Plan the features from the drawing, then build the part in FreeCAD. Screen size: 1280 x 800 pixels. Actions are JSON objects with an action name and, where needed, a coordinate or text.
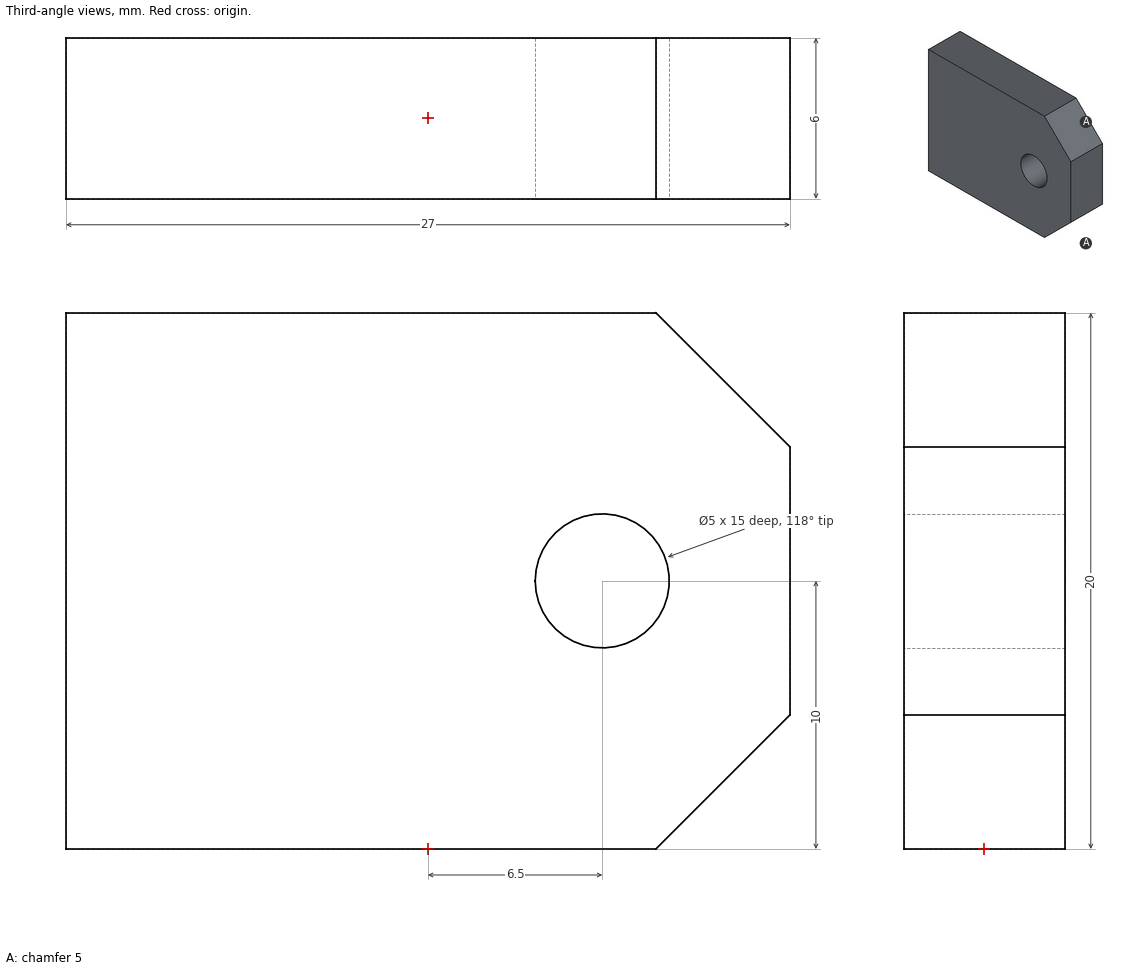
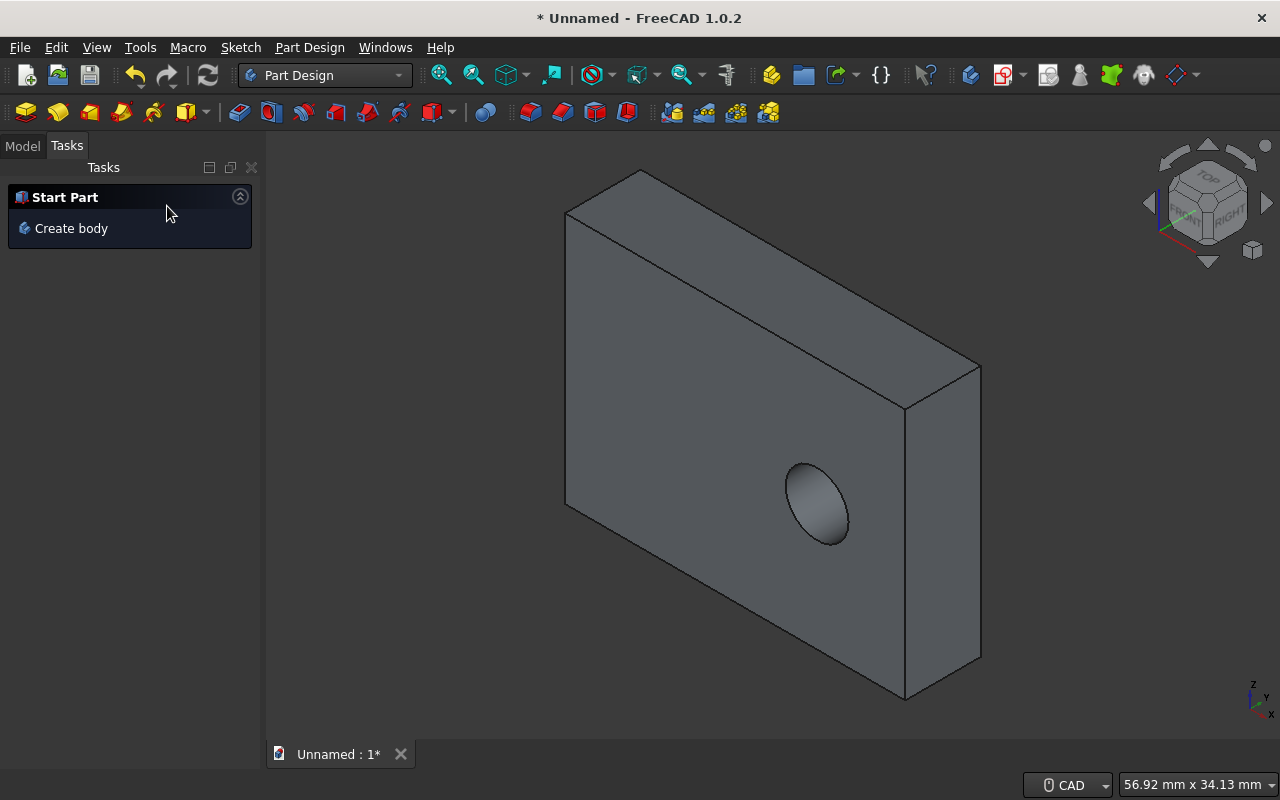
{"action": "left_click", "coordinate": [943, 387]}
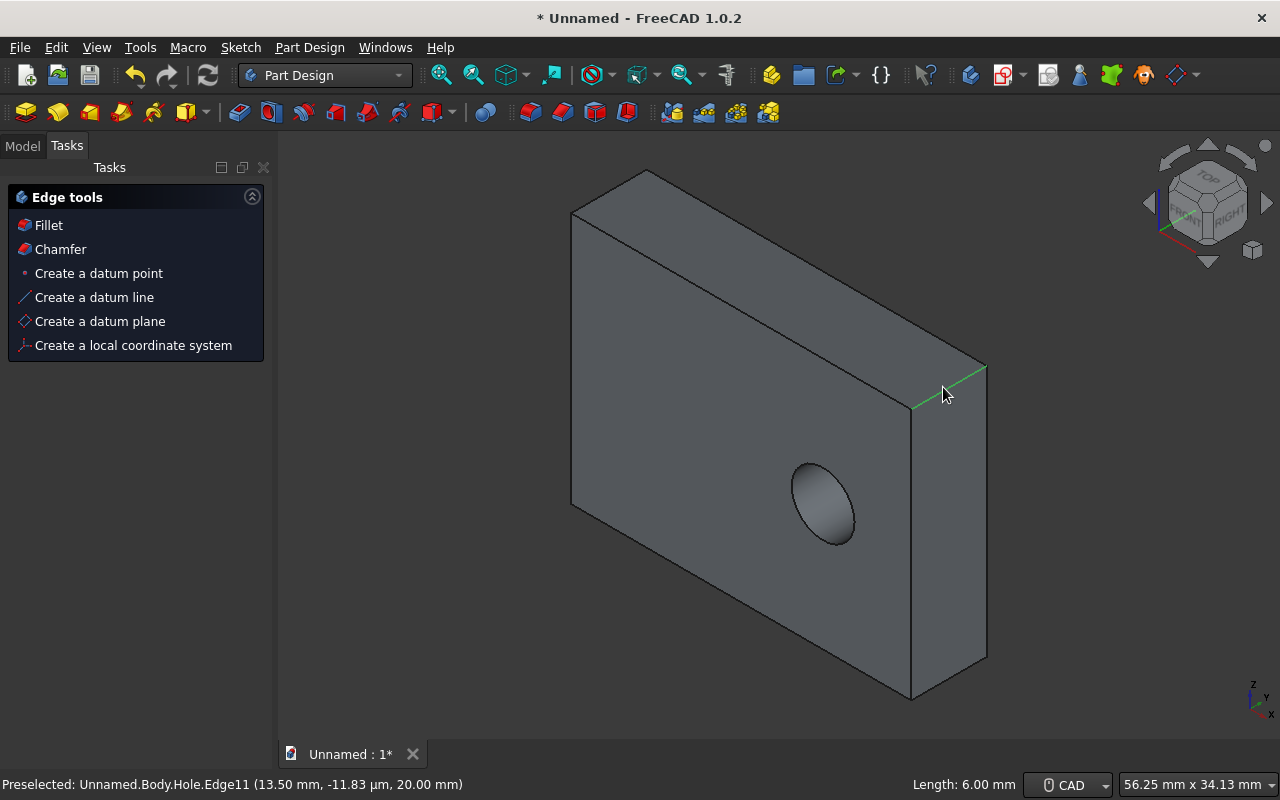
{"action": "key", "text": "2"}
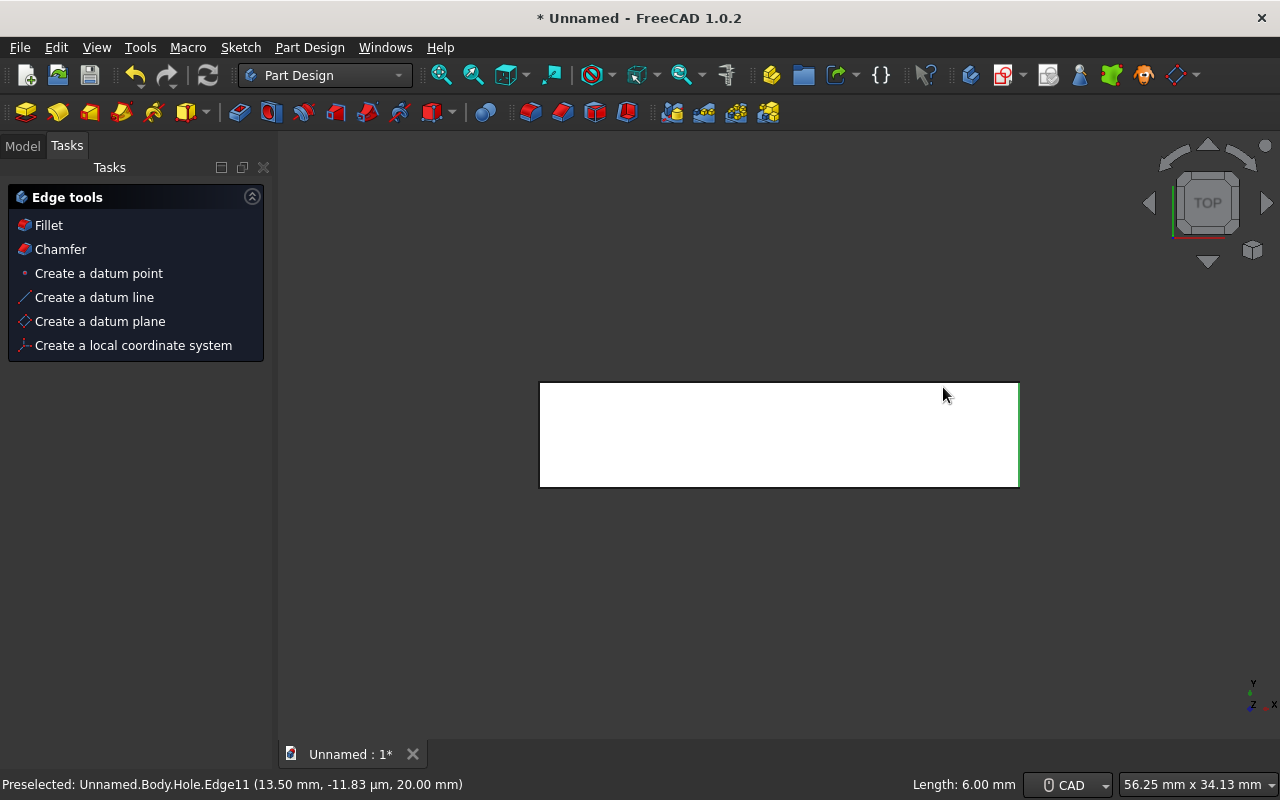
{"action": "key", "text": "1"}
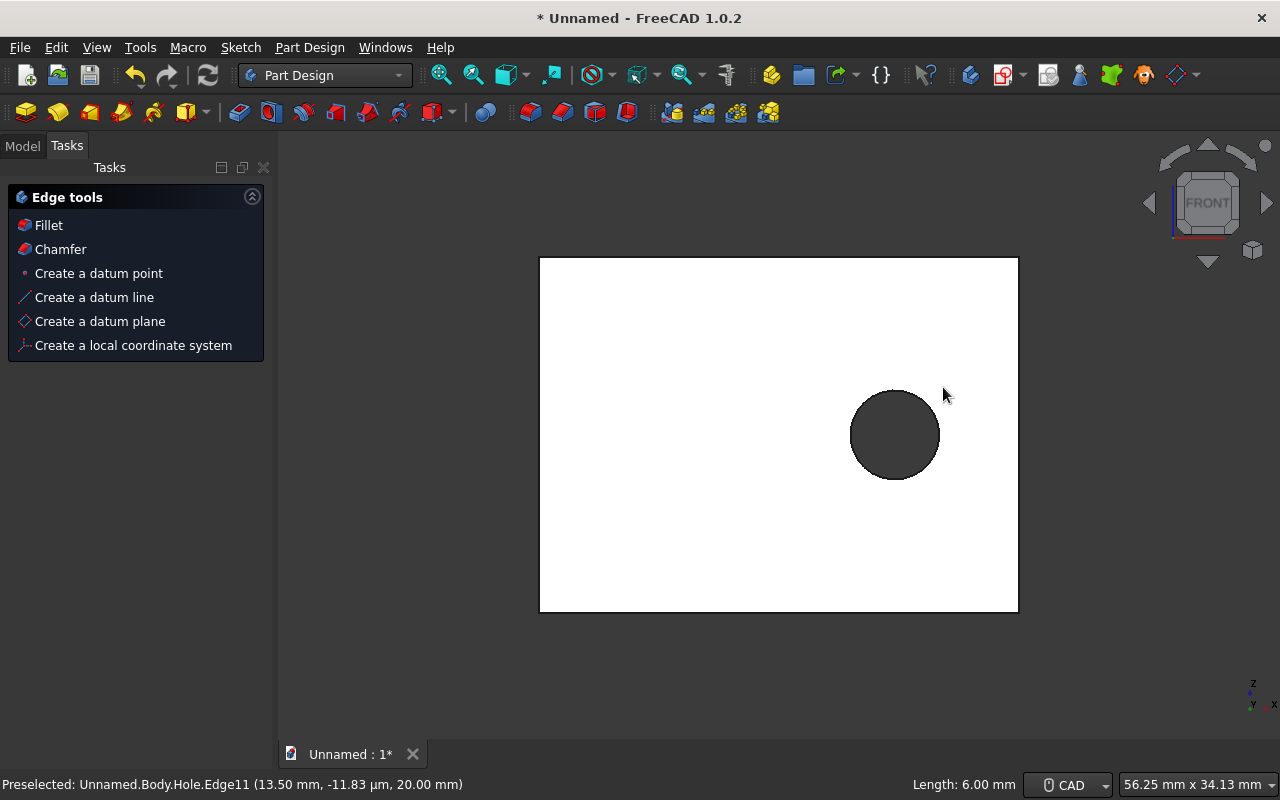
{"action": "key", "text": "3"}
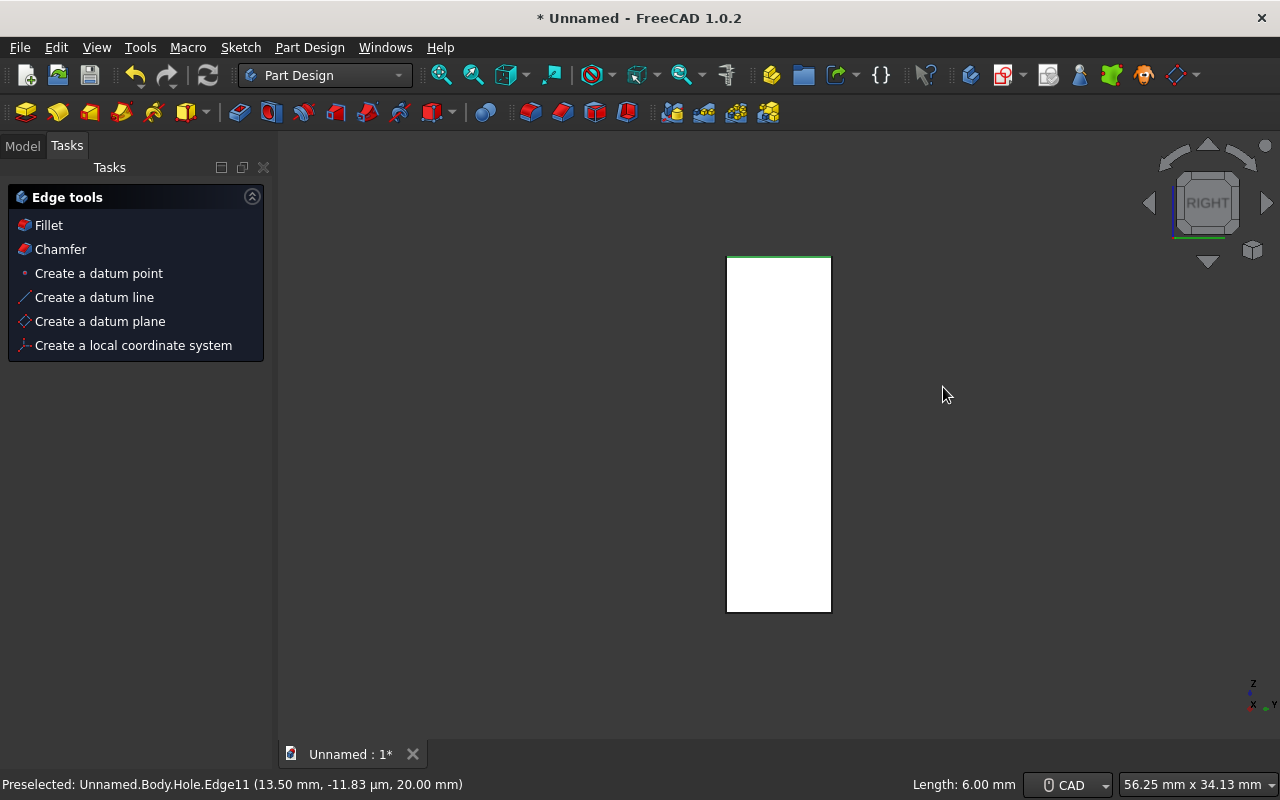
{"action": "left_click", "coordinate": [779, 612], "text": "ctrl"}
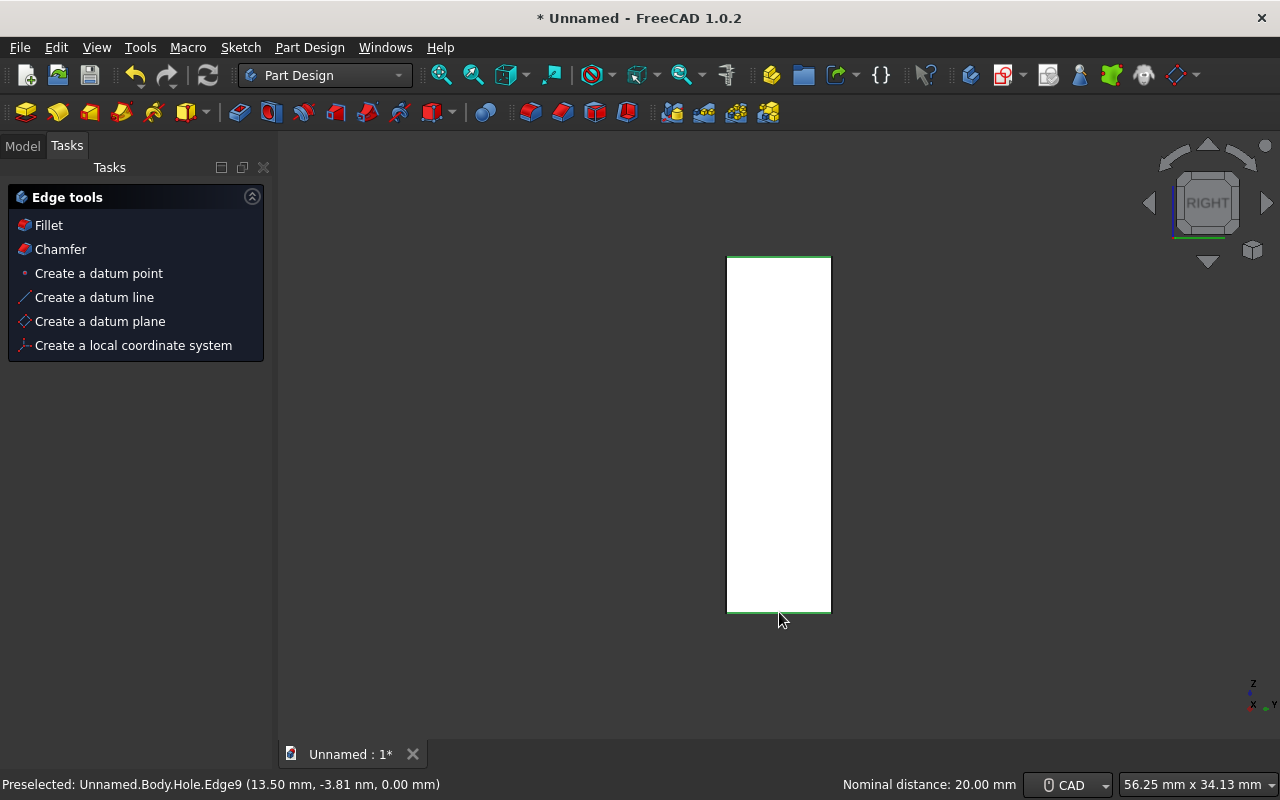
{"action": "left_click", "coordinate": [564, 112]}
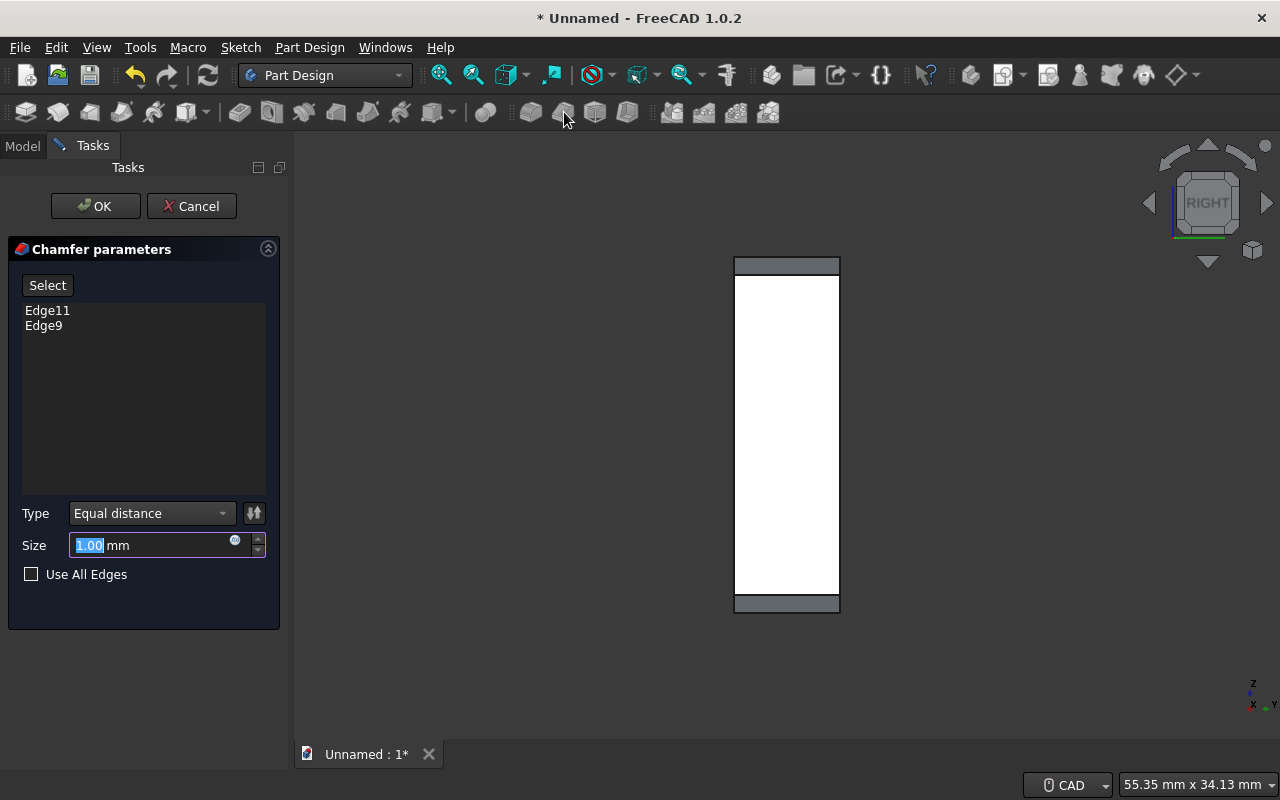
{"action": "type", "text": "5"}
{"action": "key", "text": "Tab"}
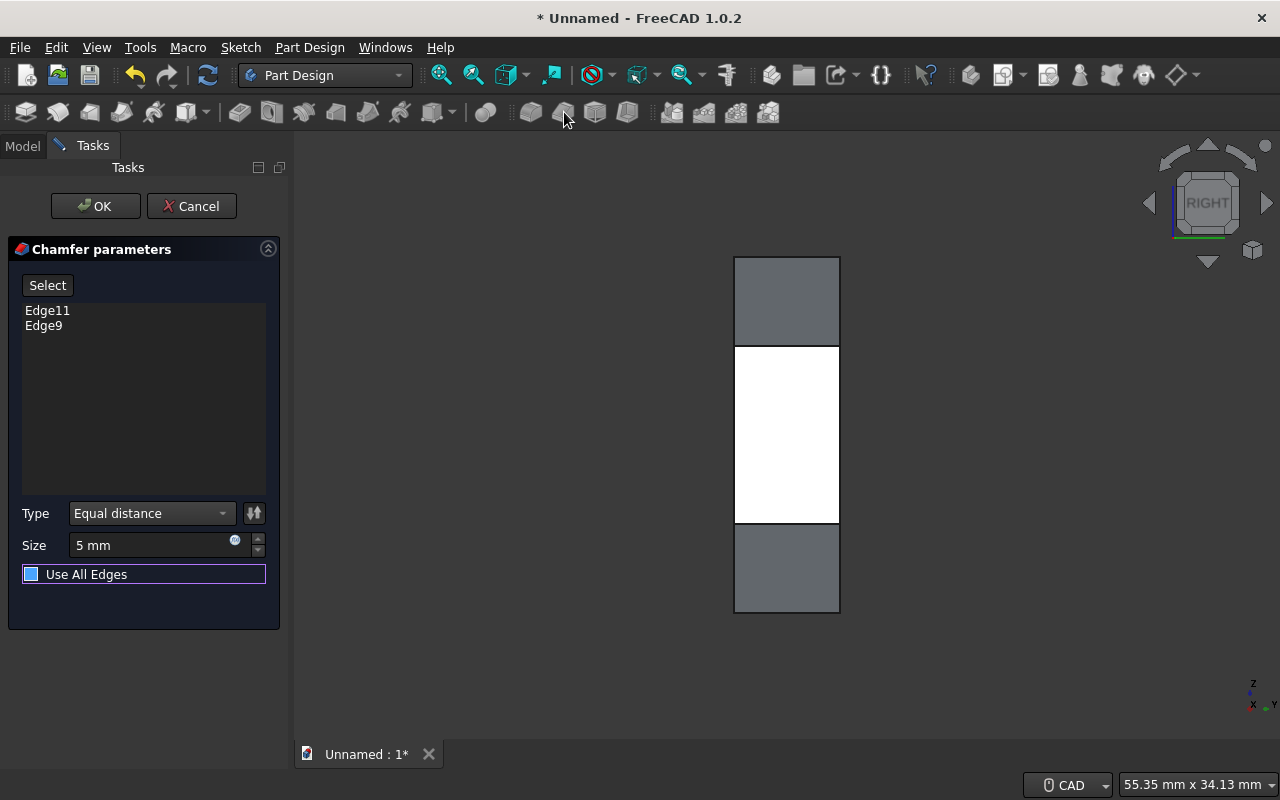
{"action": "left_click", "coordinate": [96, 206]}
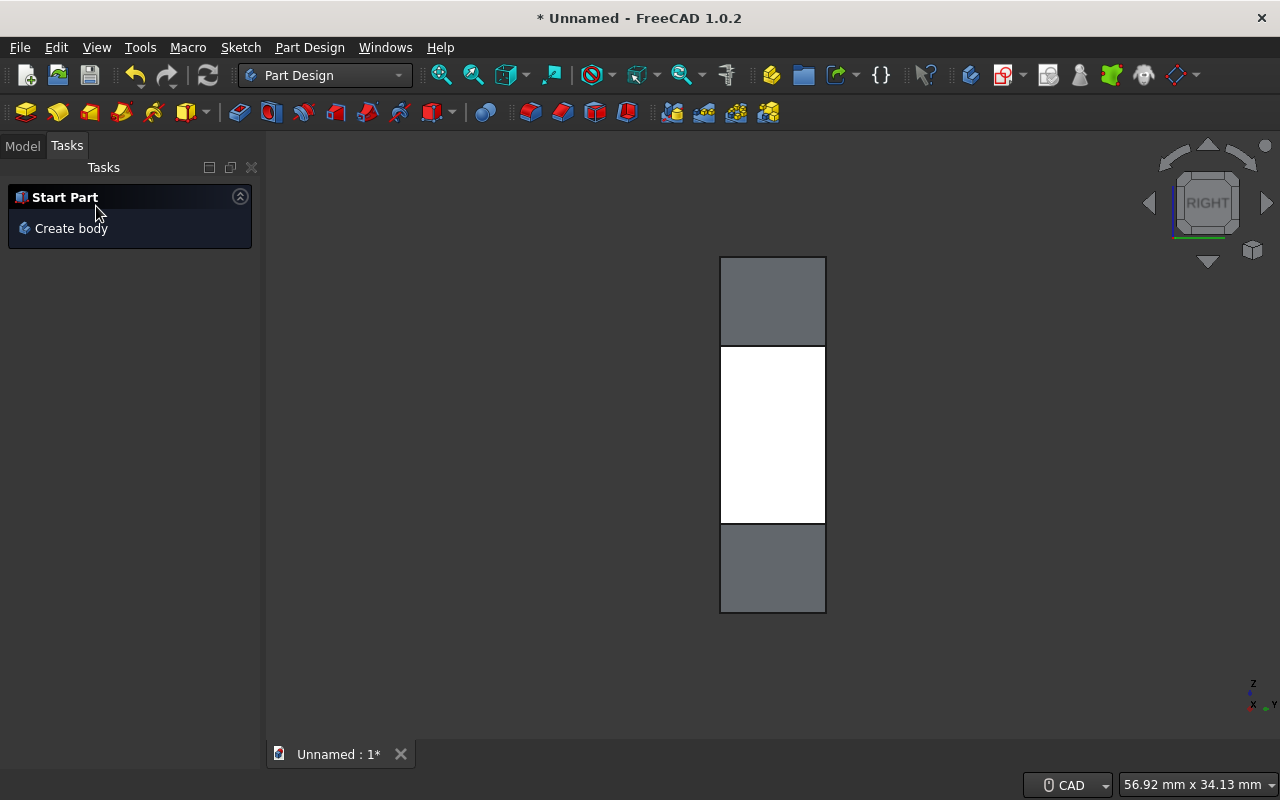
{"action": "key", "text": "0"}